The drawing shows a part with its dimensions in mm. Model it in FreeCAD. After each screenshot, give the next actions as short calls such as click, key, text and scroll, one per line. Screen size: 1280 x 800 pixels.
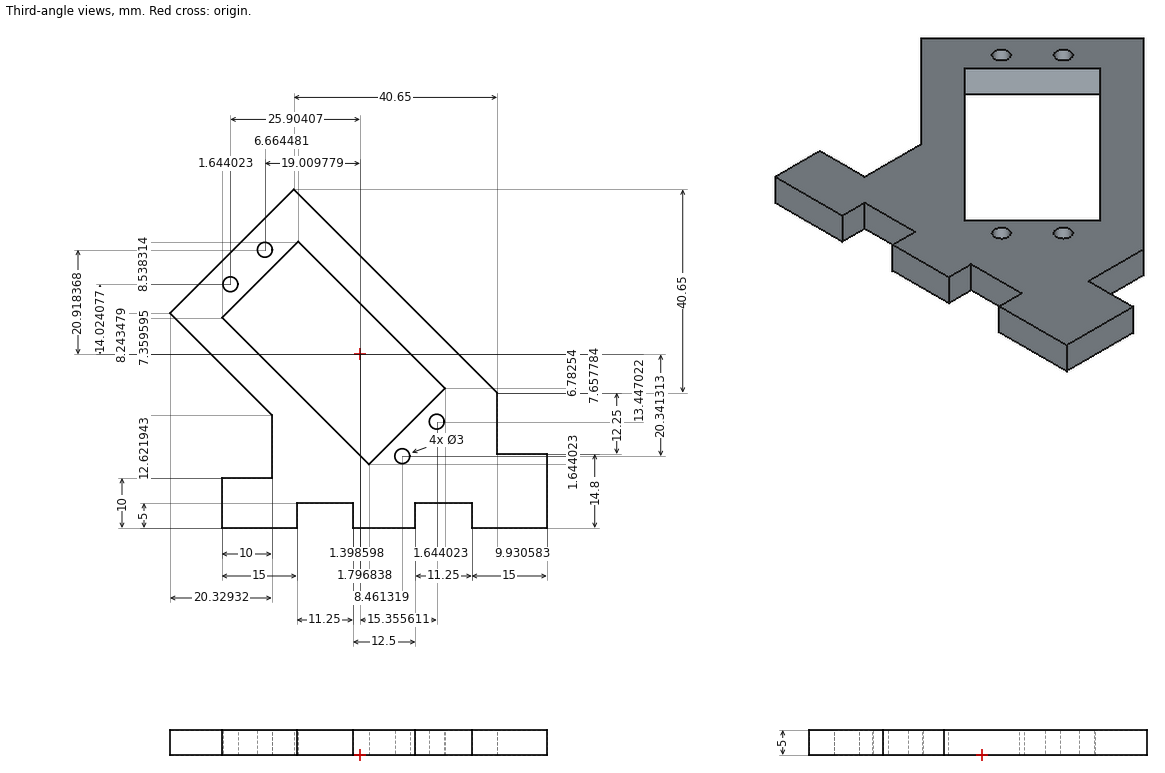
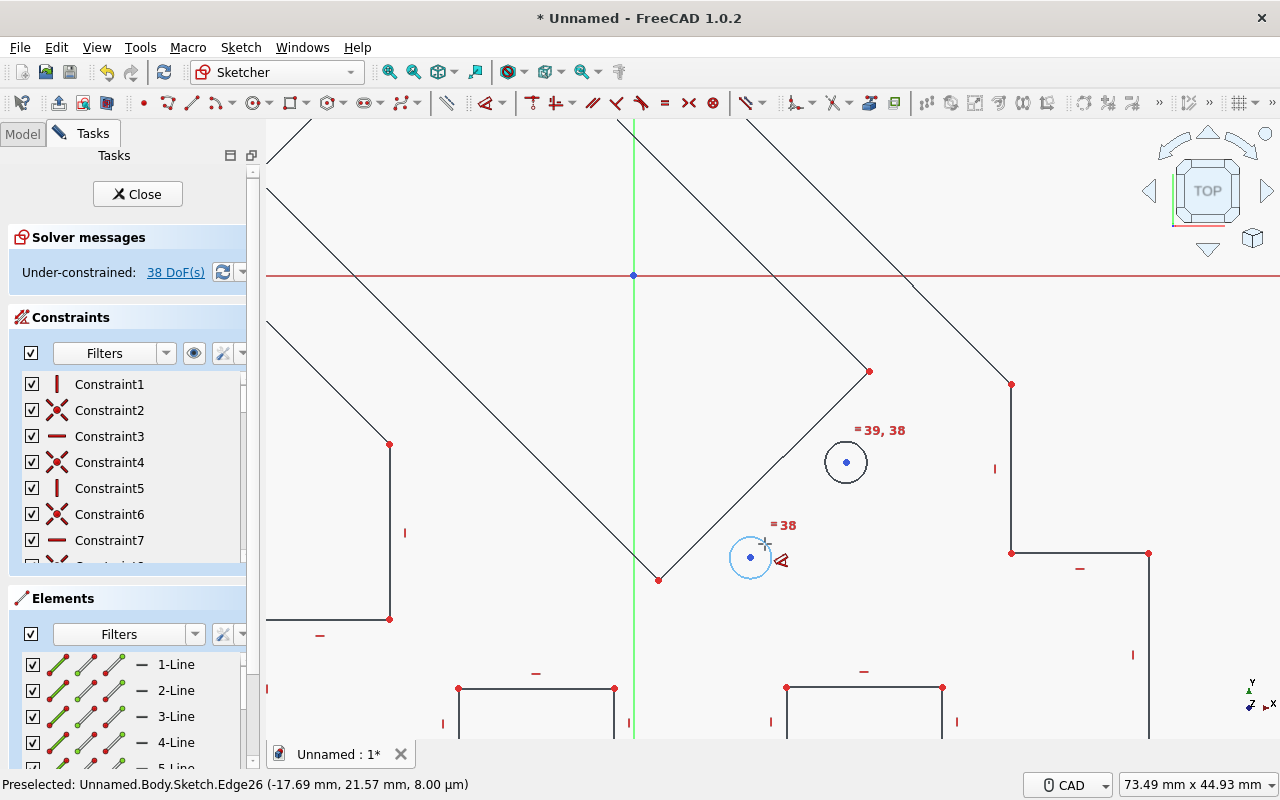
click(765, 543)
click(787, 520)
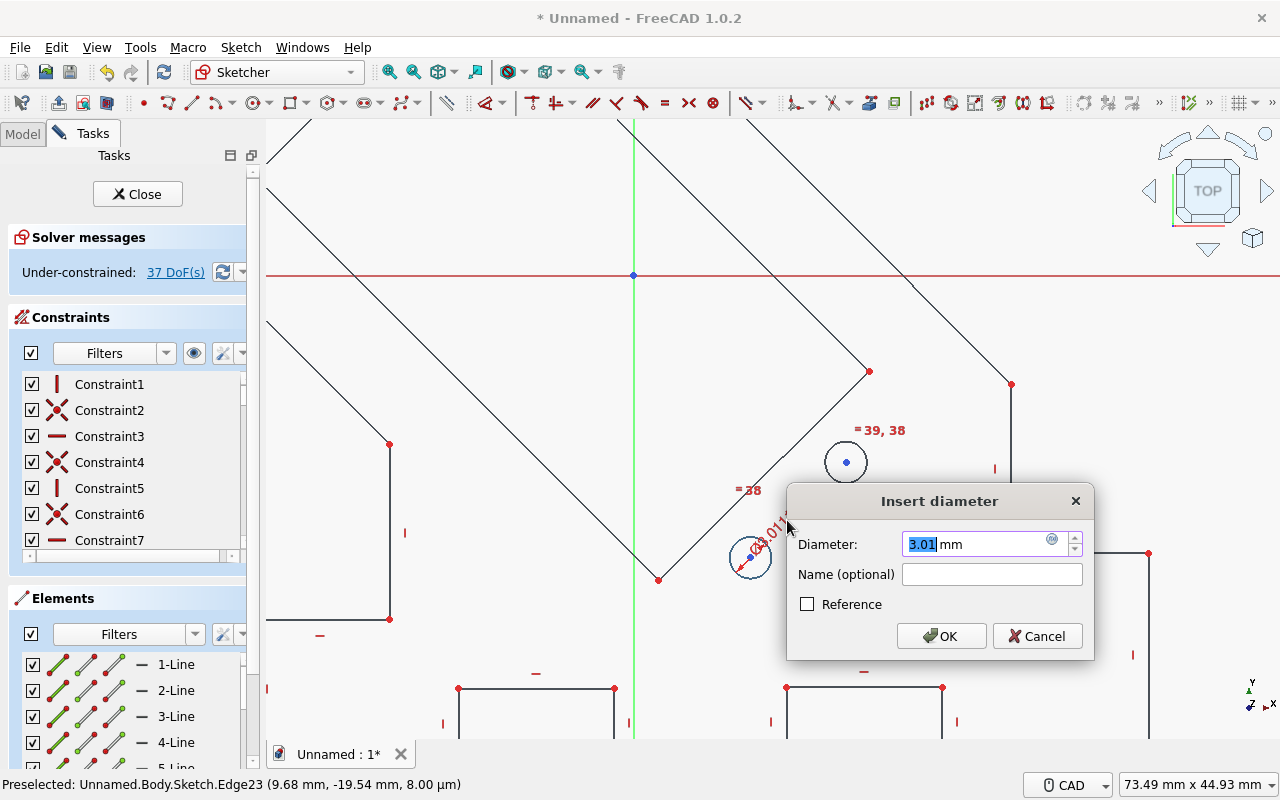
text(3)
key(Return)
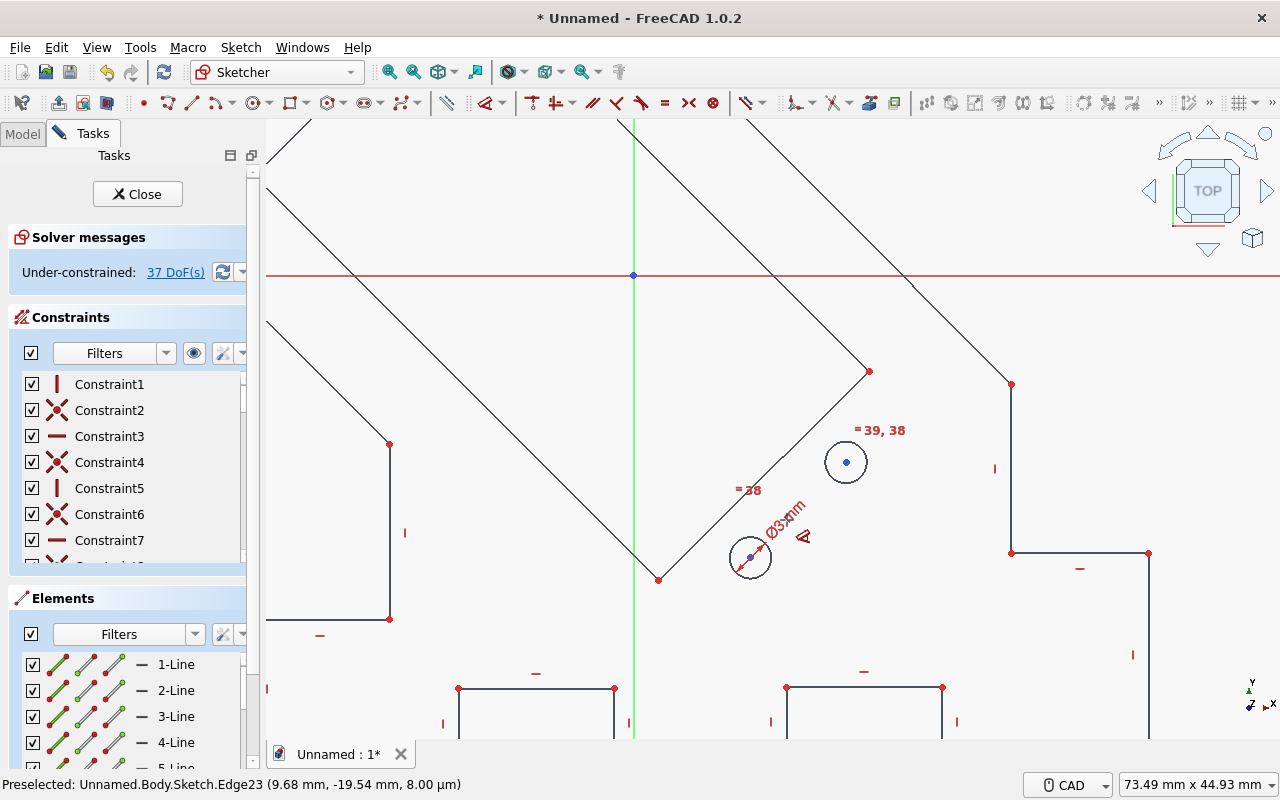
click(459, 709)
click(425, 700)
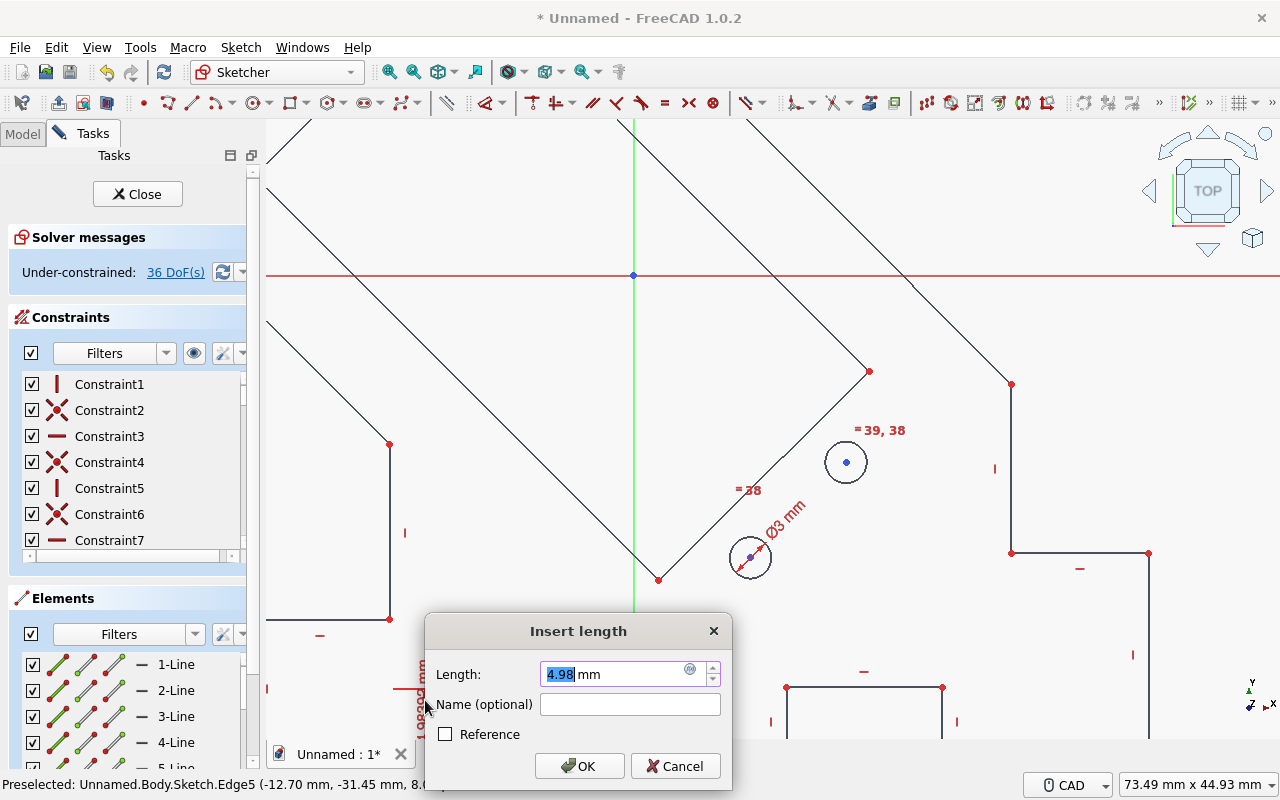
text(5)
key(Return)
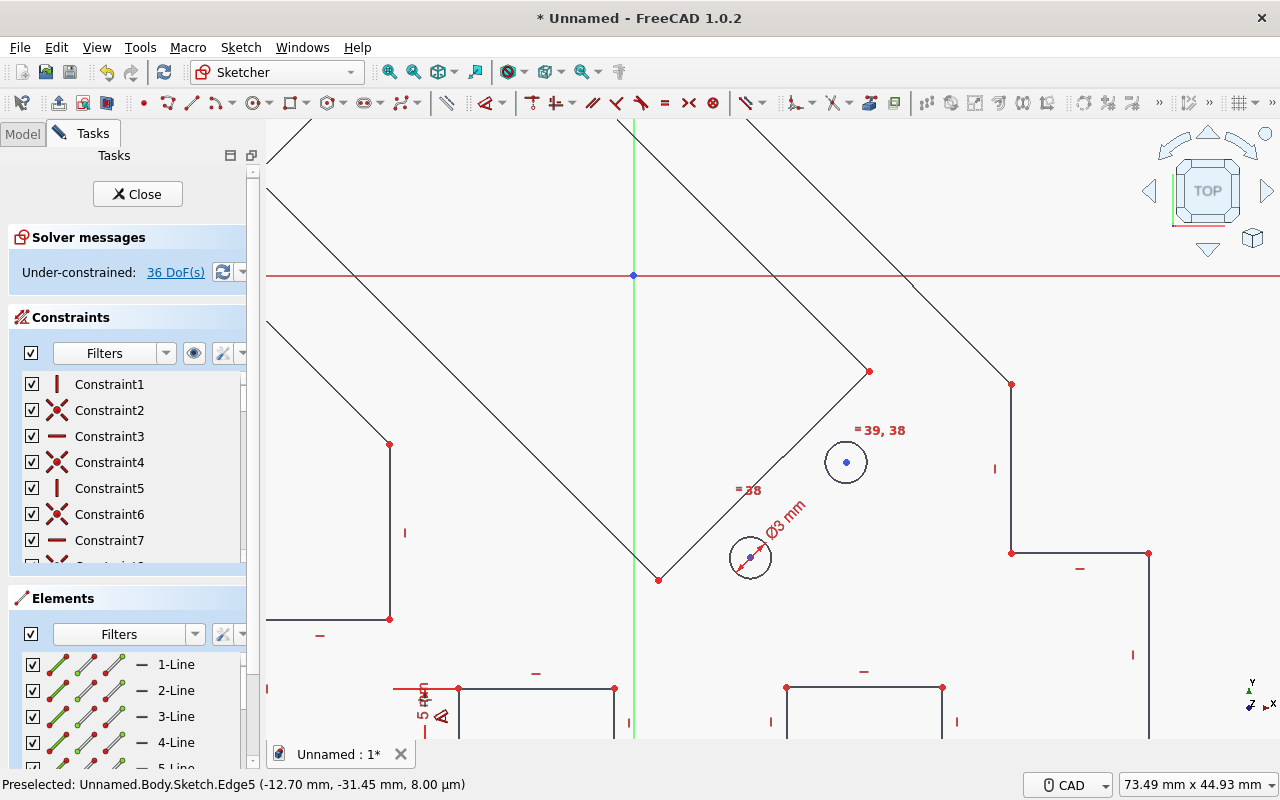
click(614, 709)
click(580, 705)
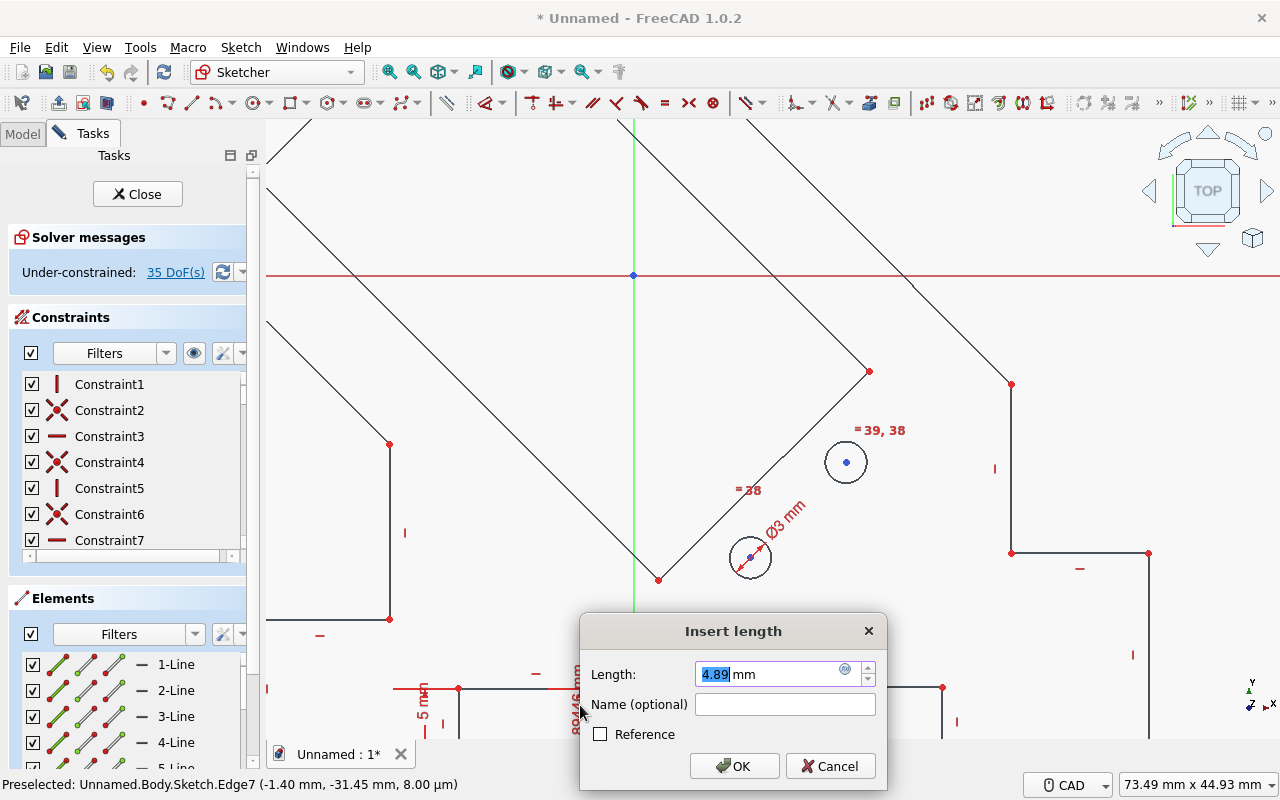
text(5)
key(Return)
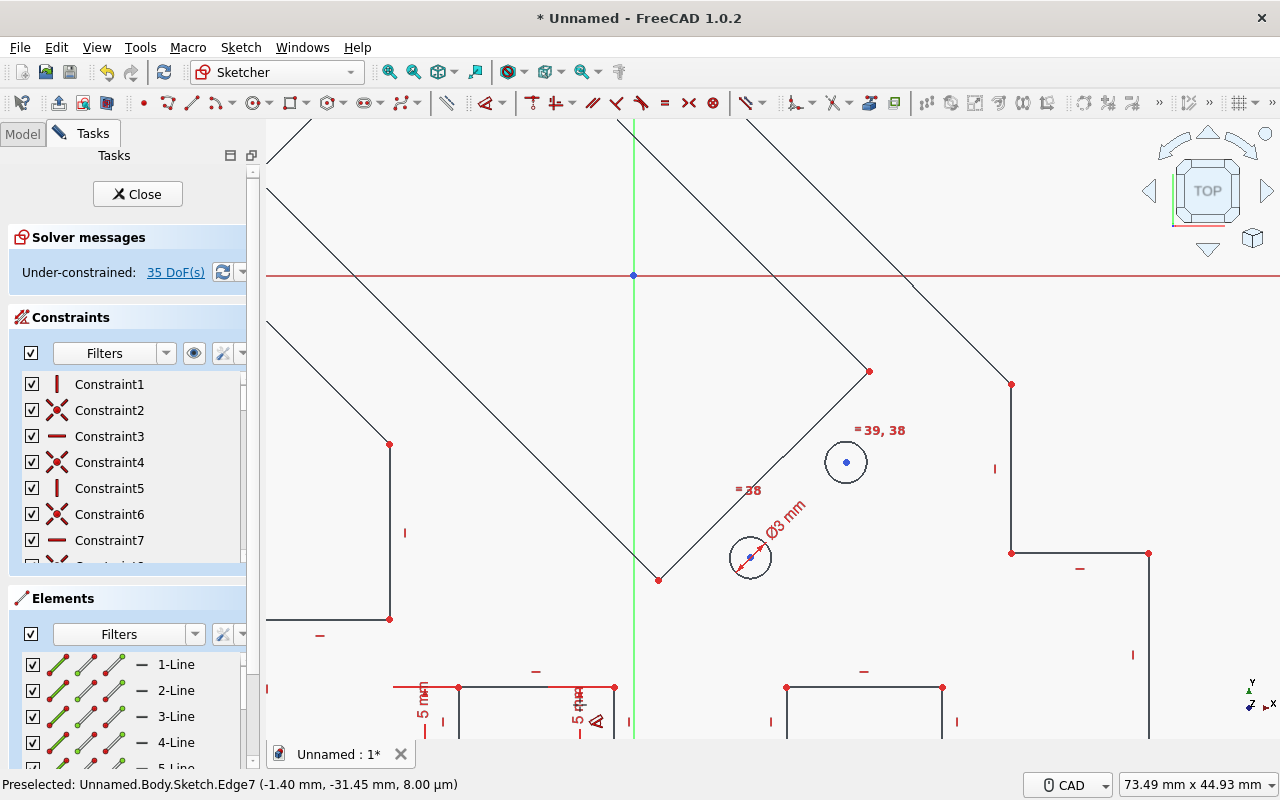
click(787, 708)
click(821, 705)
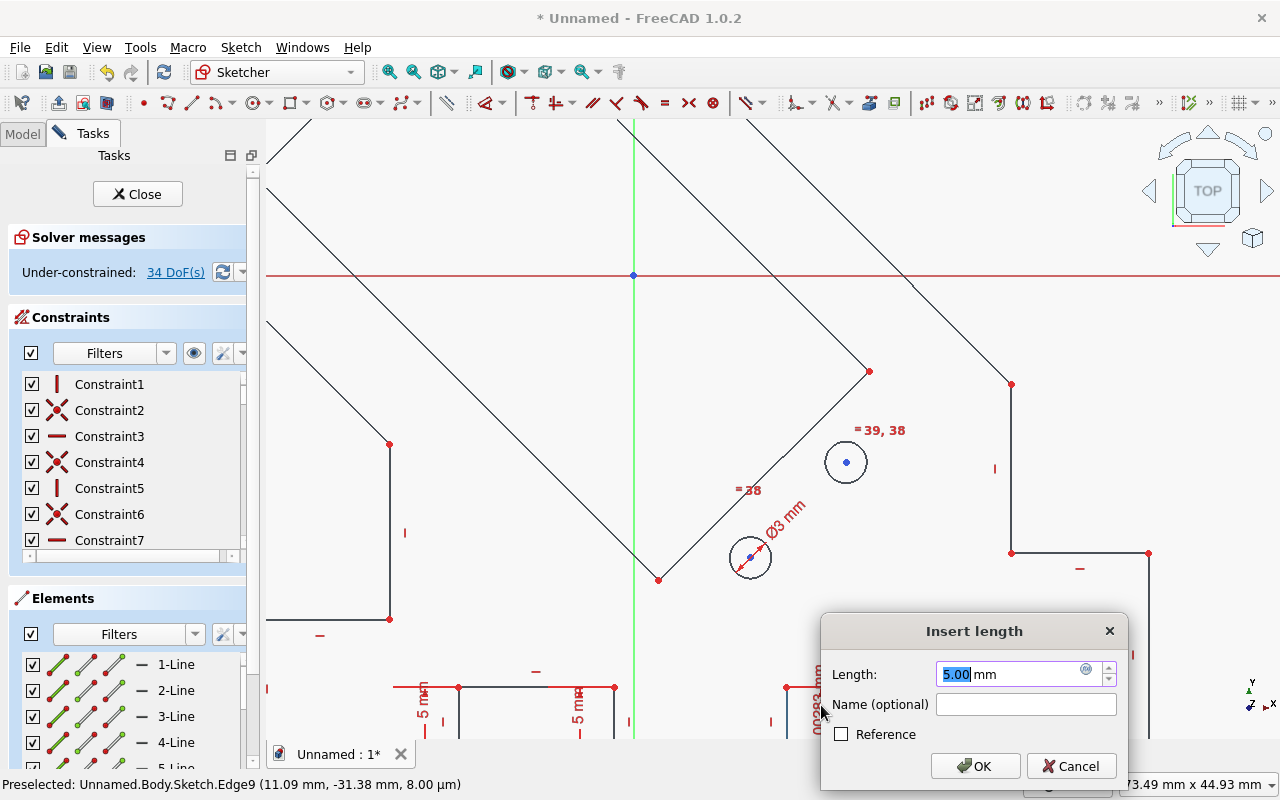
text(5)
key(Return)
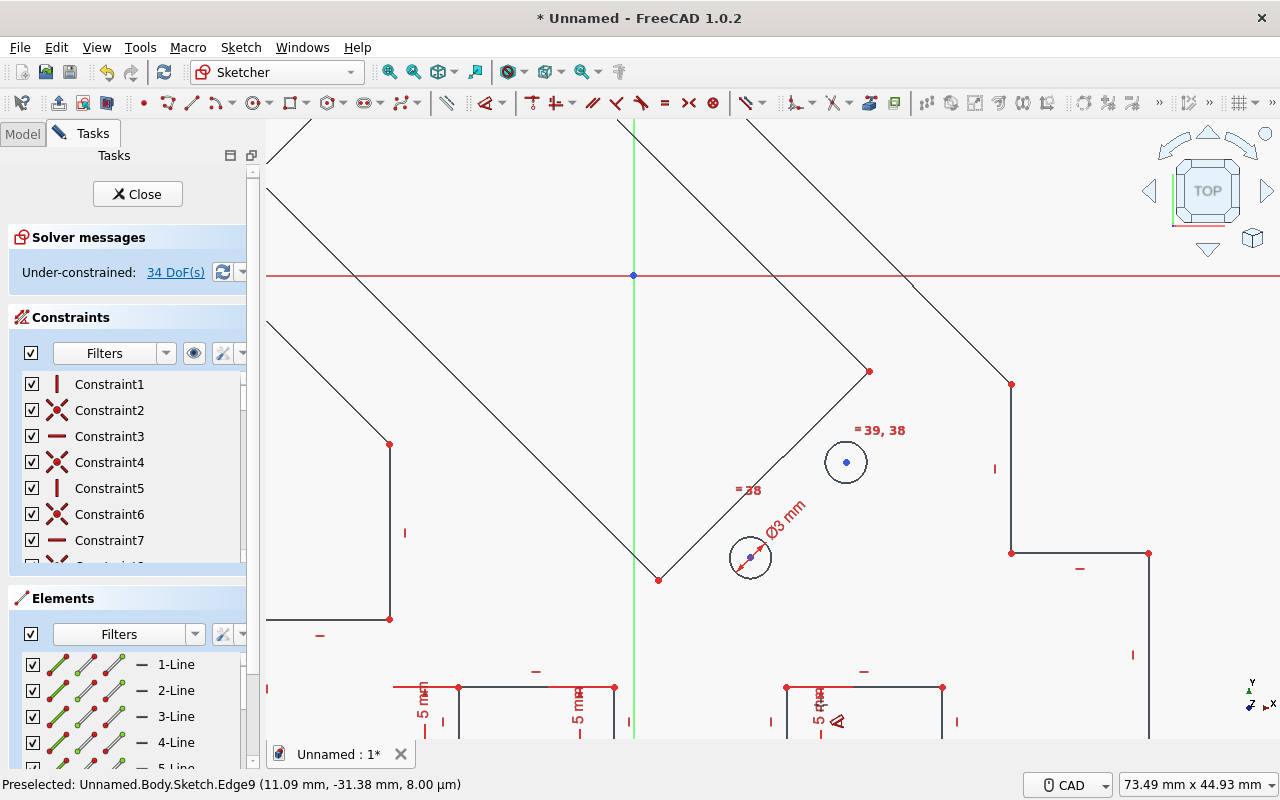
click(942, 708)
click(976, 699)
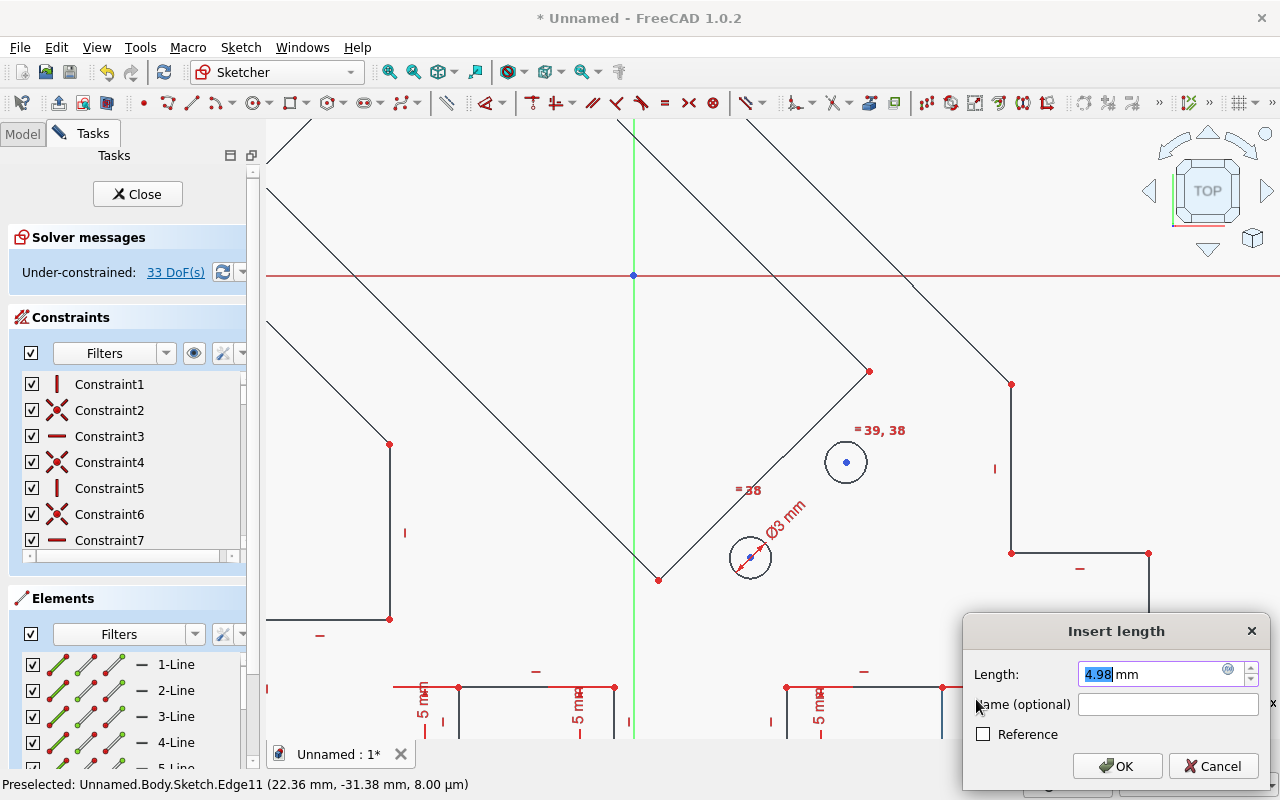
text(5)
key(Return)